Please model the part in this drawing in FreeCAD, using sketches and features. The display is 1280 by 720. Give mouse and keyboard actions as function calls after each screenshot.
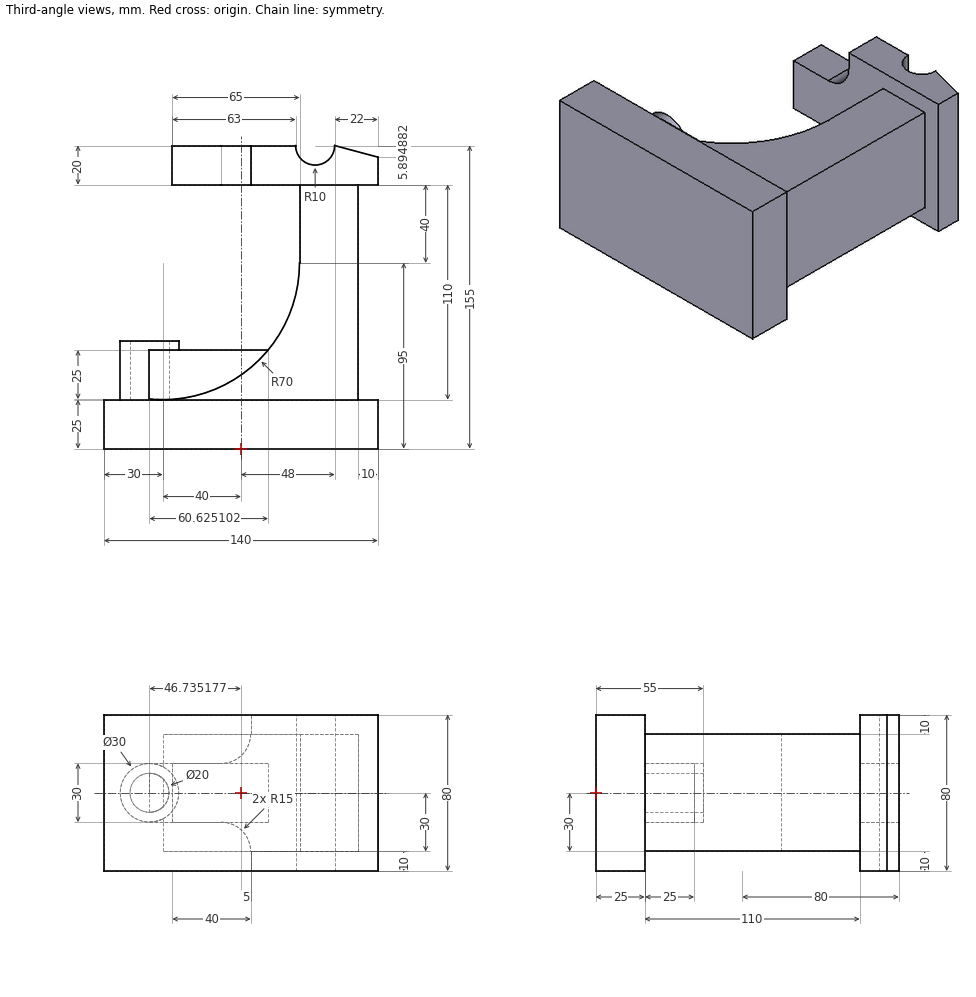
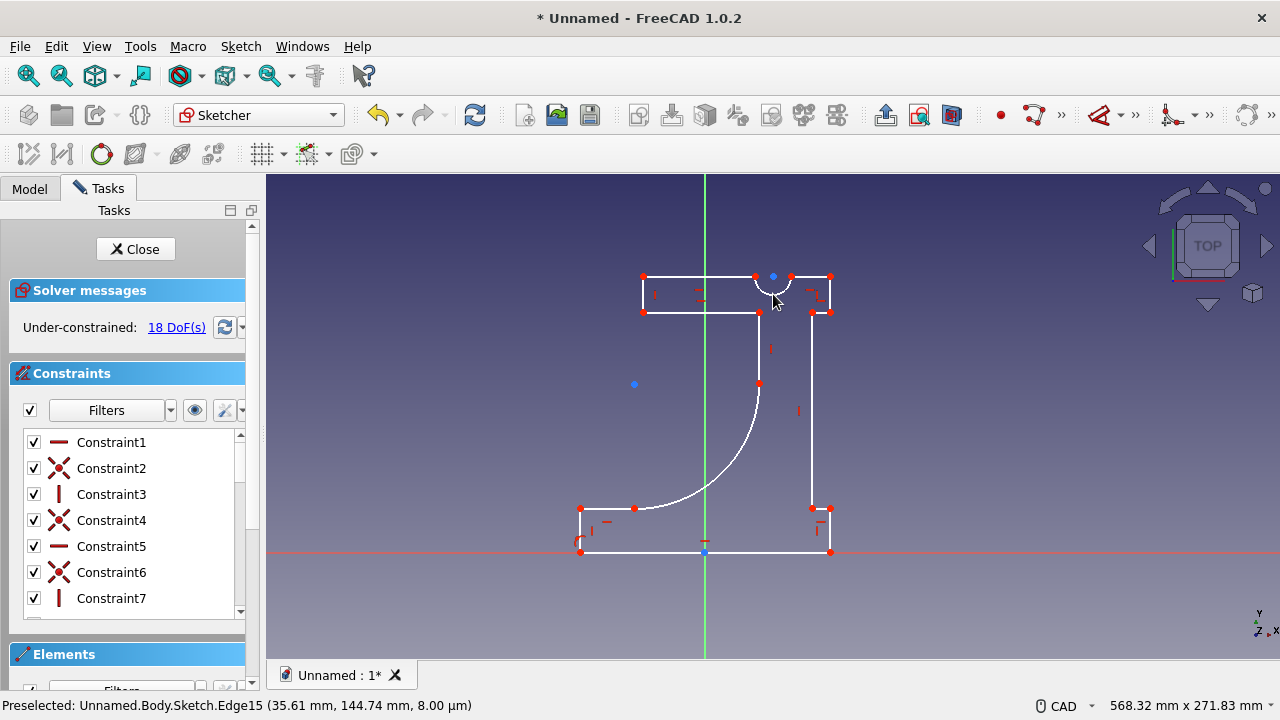
click(580, 509)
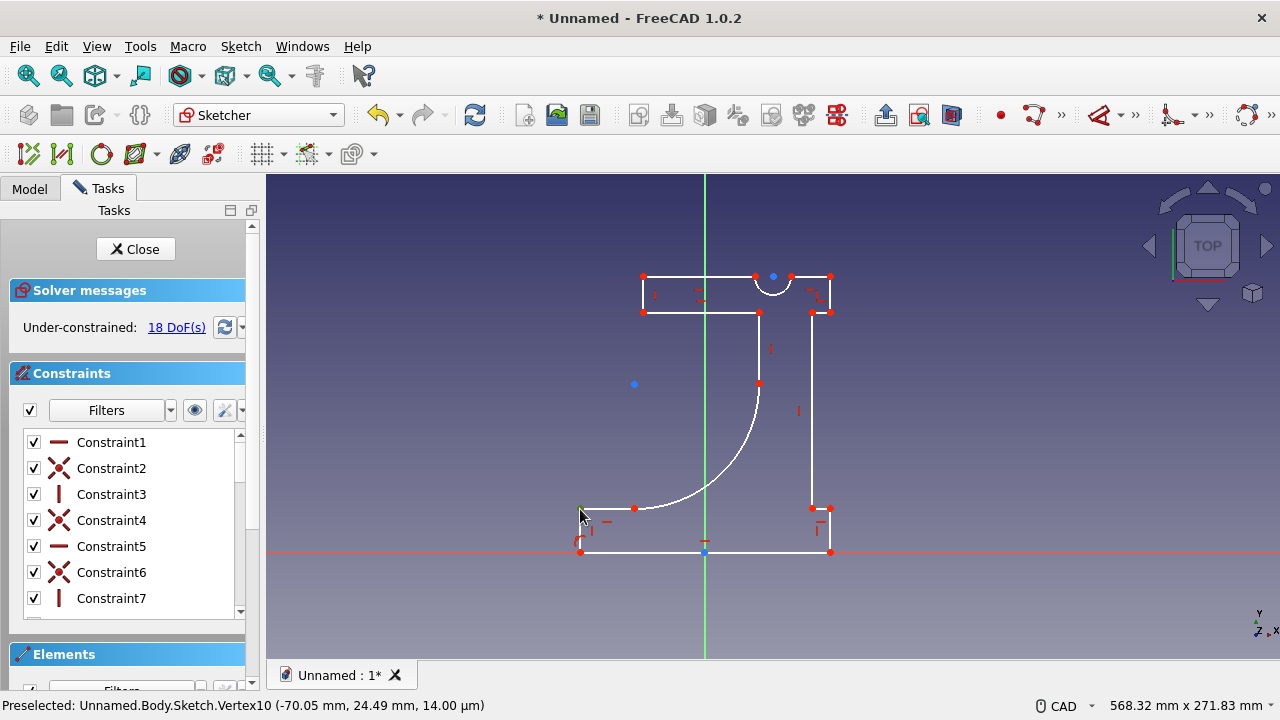
click(830, 509)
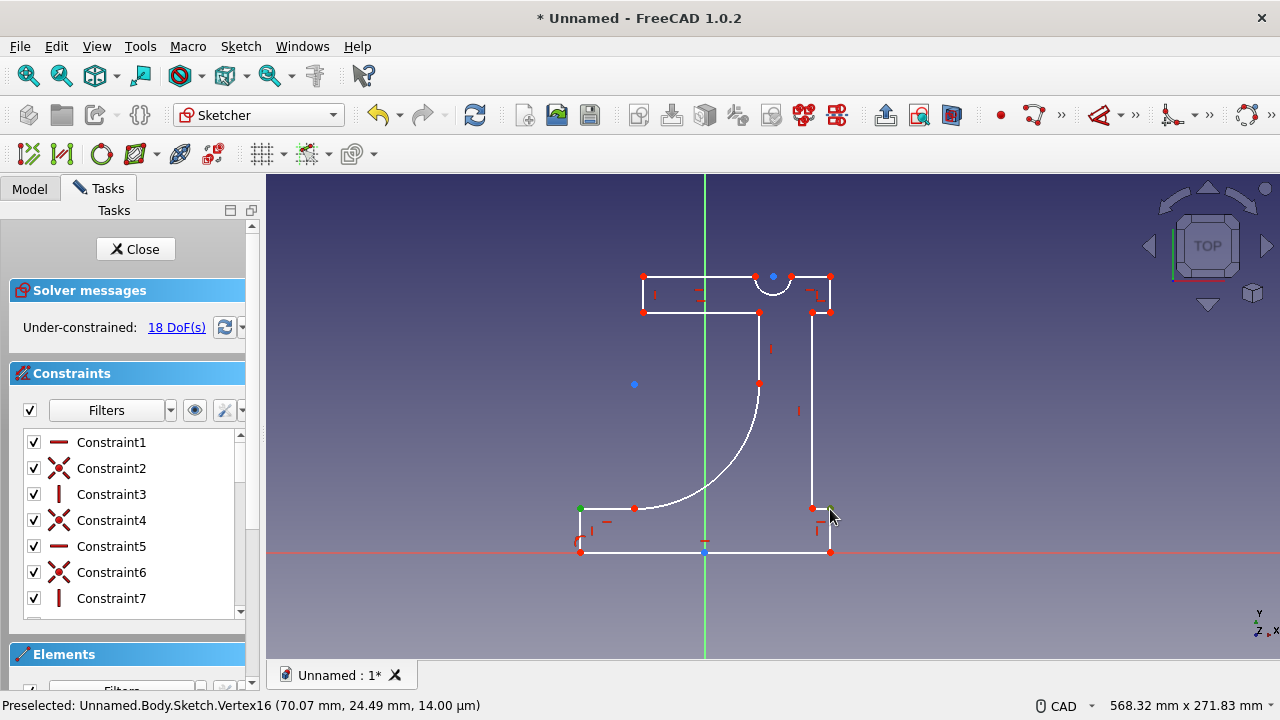
click(705, 600)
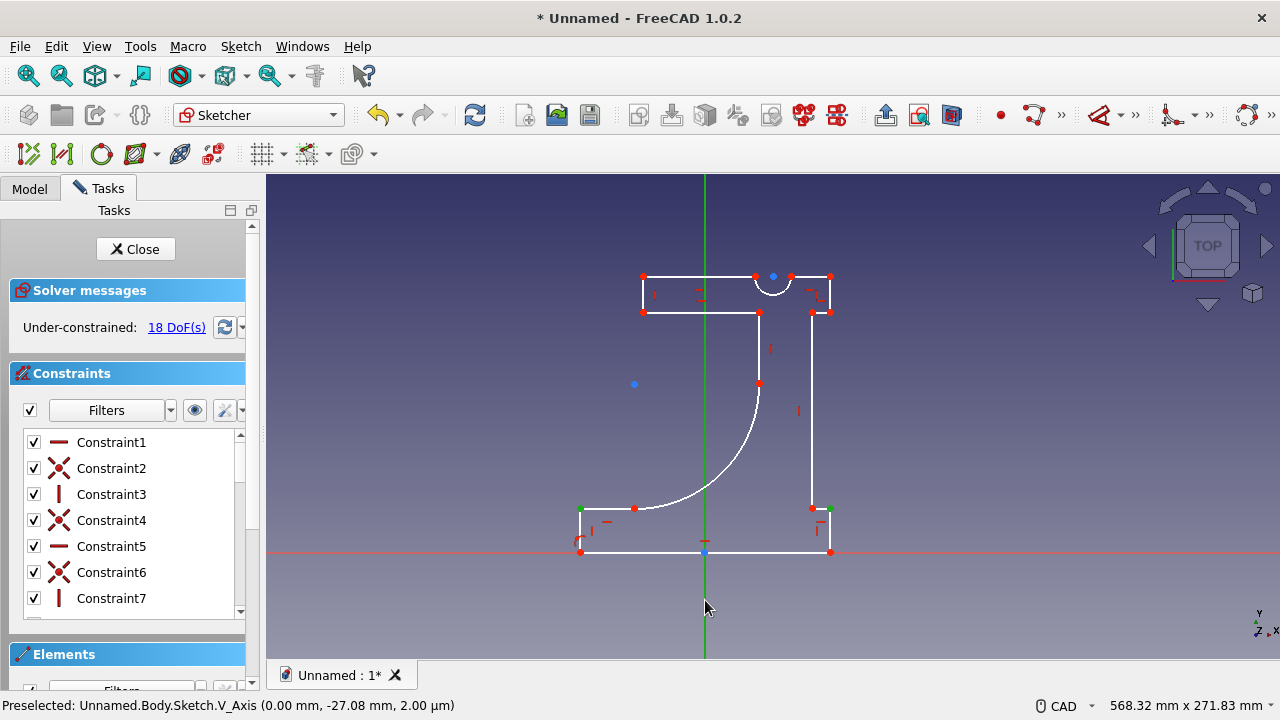
key(s)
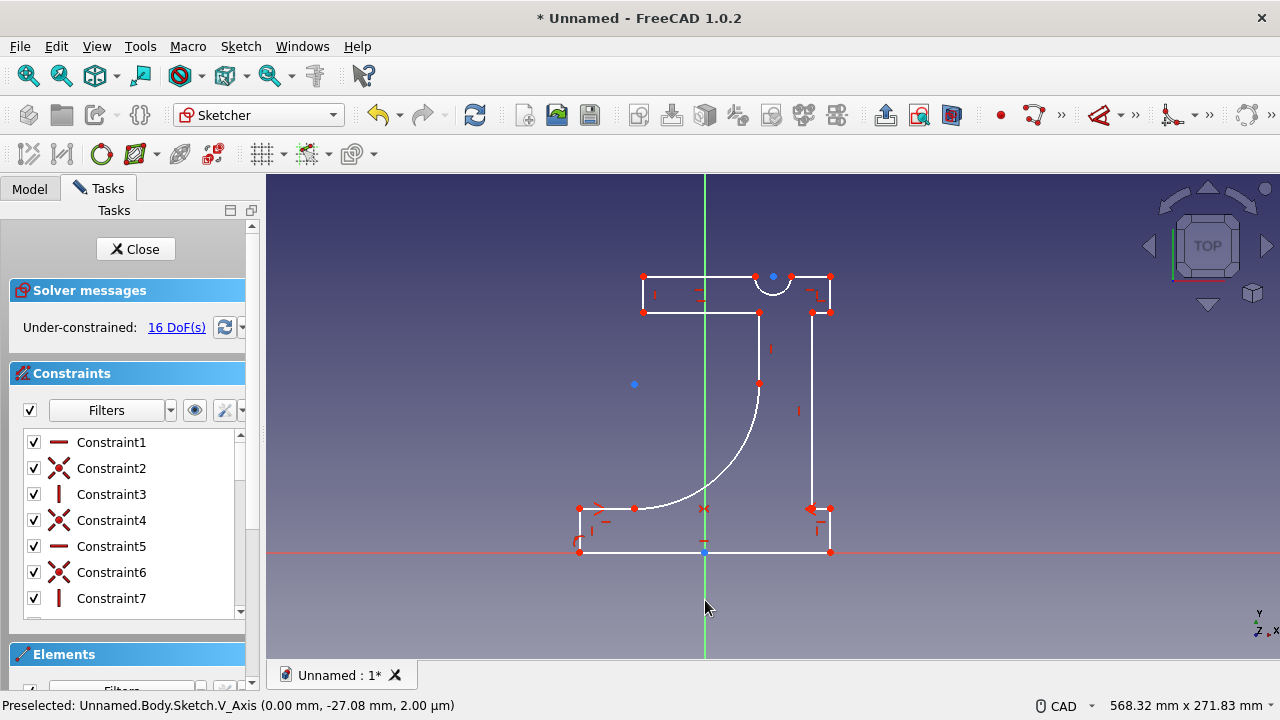
click(1098, 116)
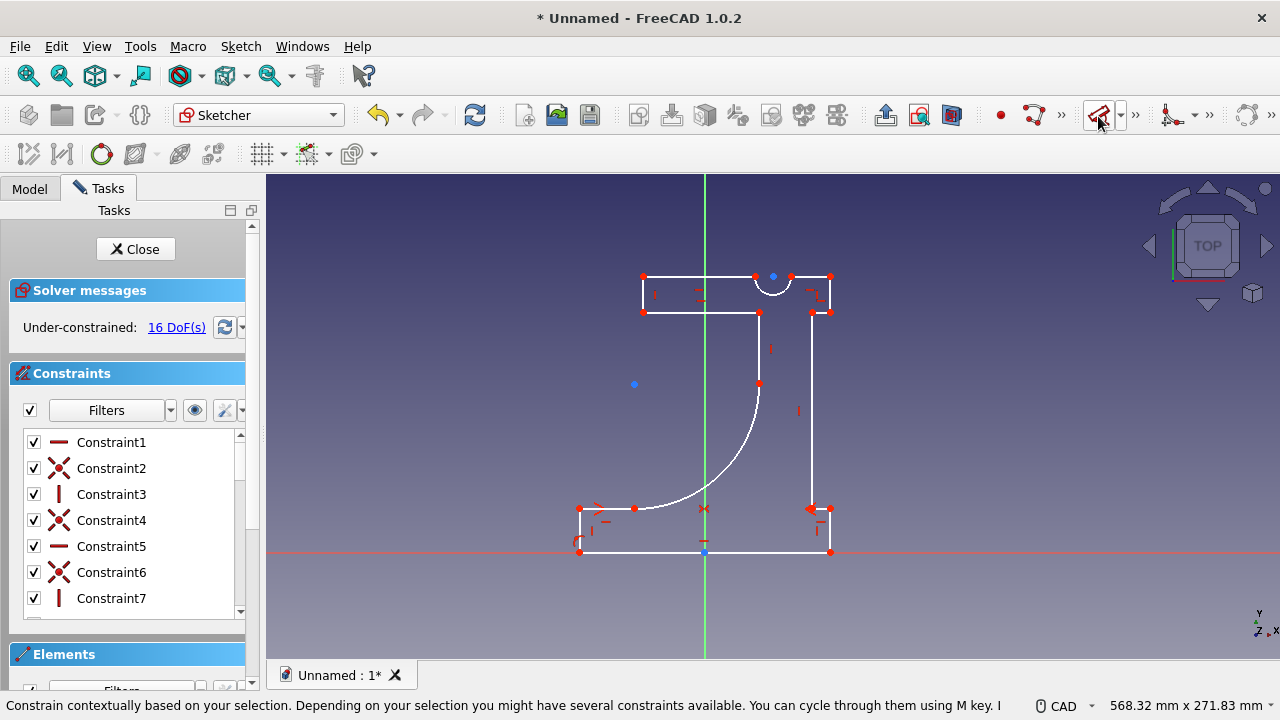
click(691, 495)
click(764, 472)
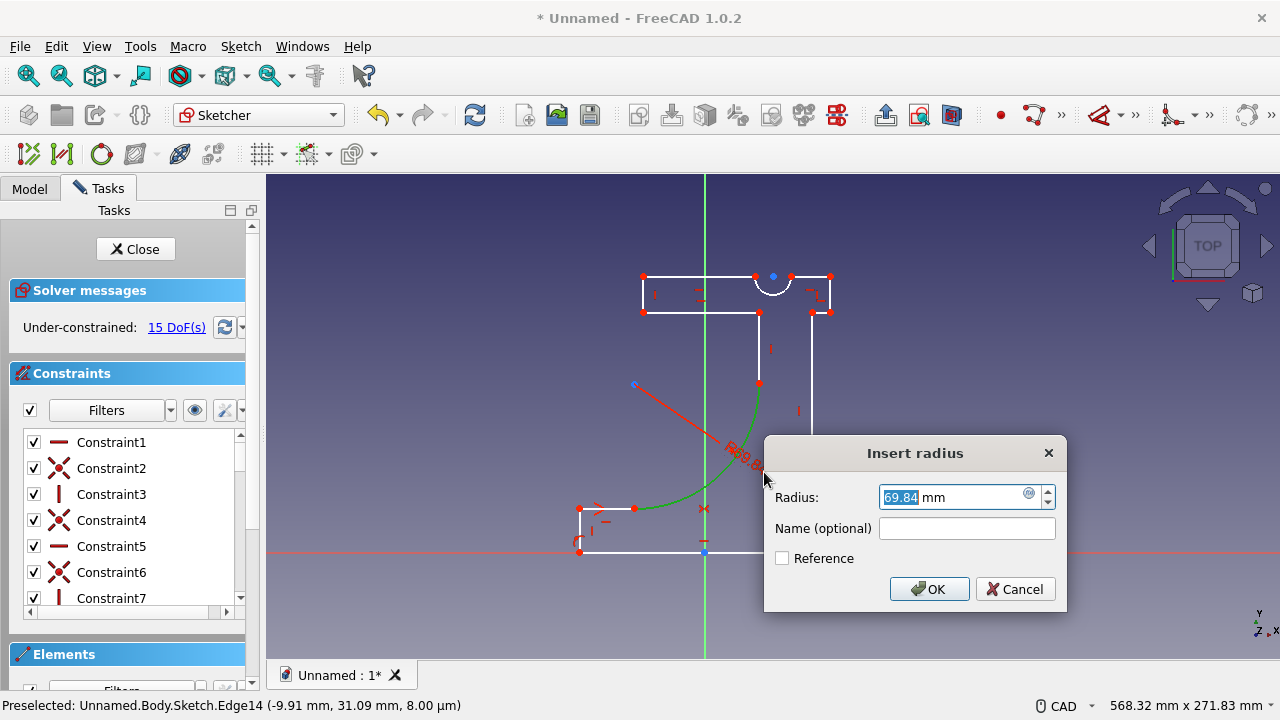
text(70)
key(Return)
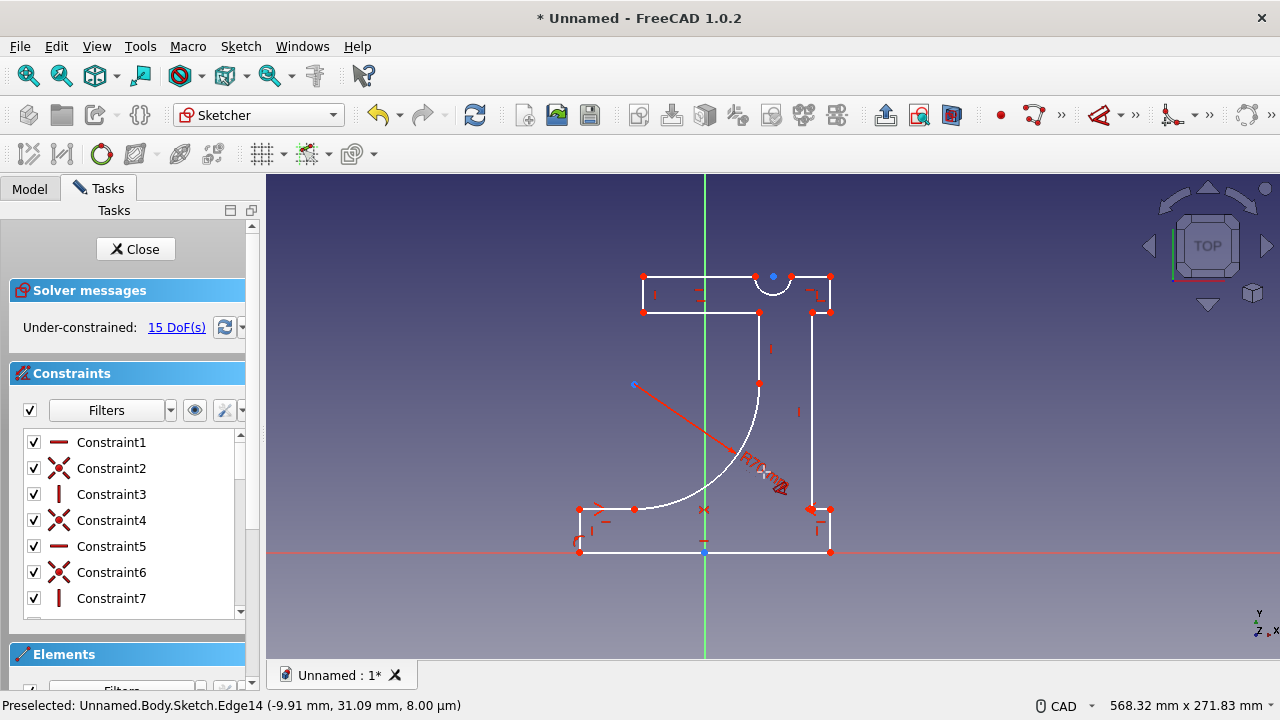
scroll(762, 292, up, 4)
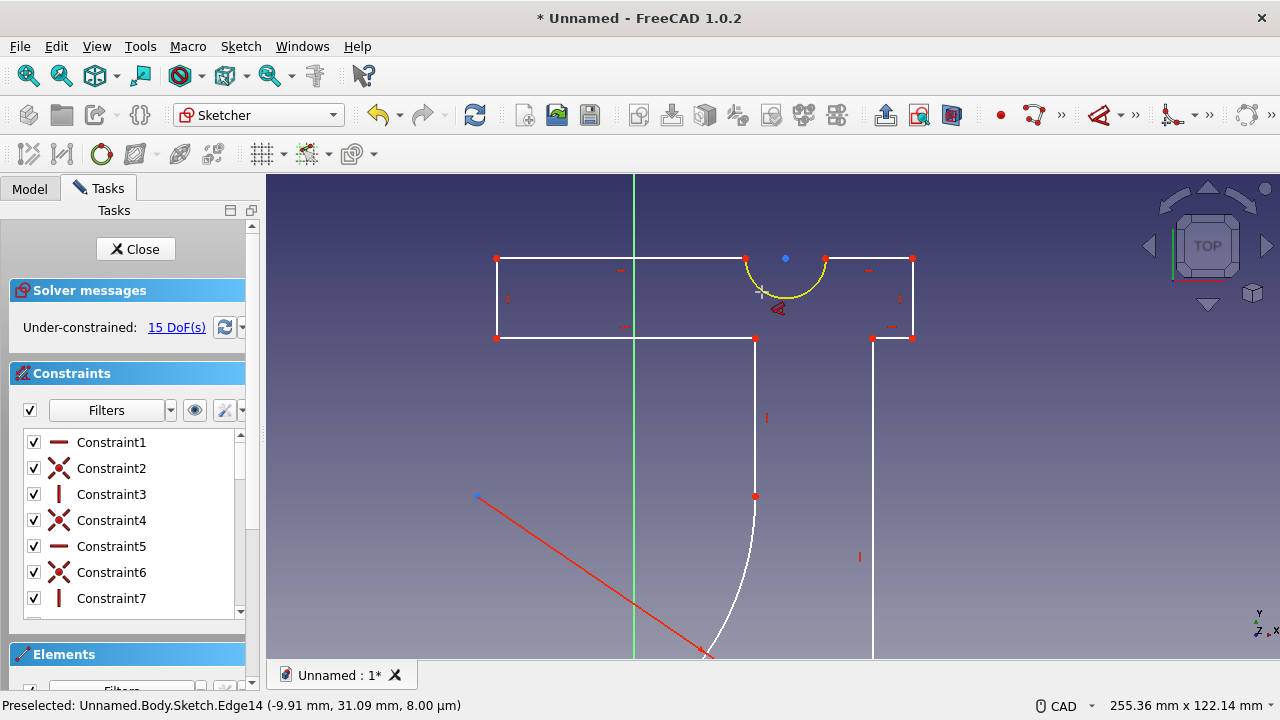
click(762, 291)
click(743, 317)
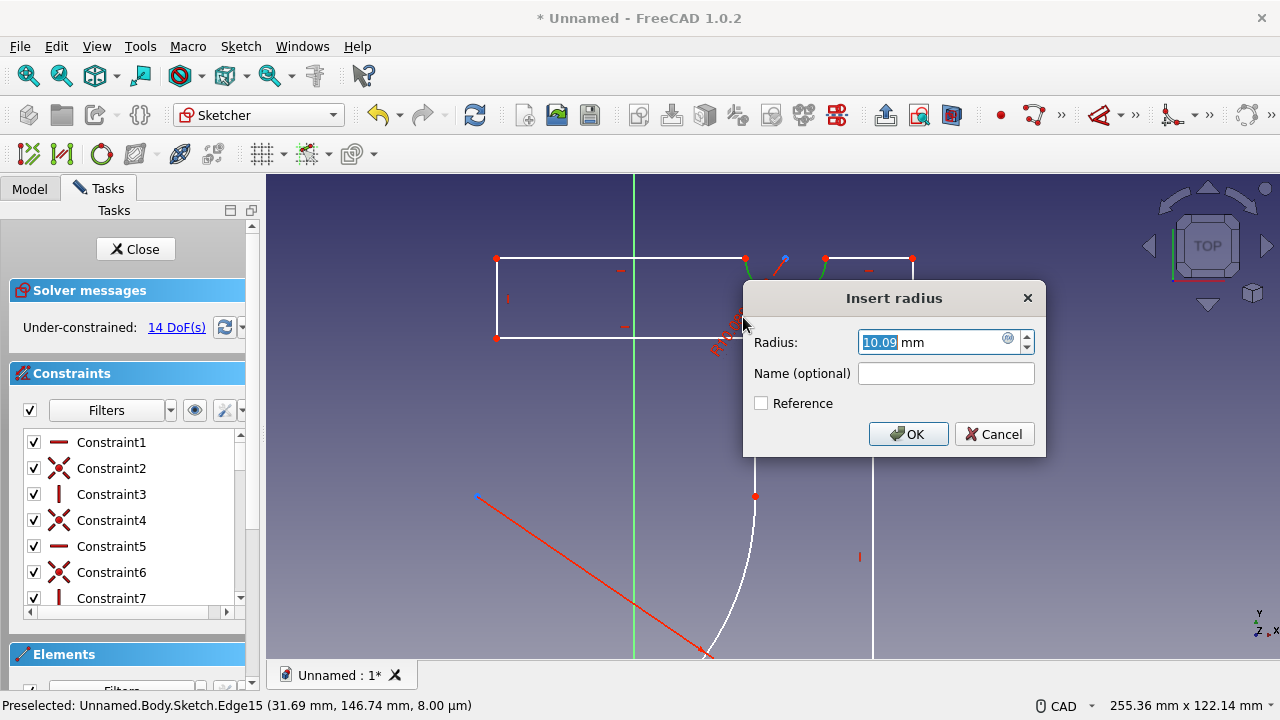
text(10)
key(Return)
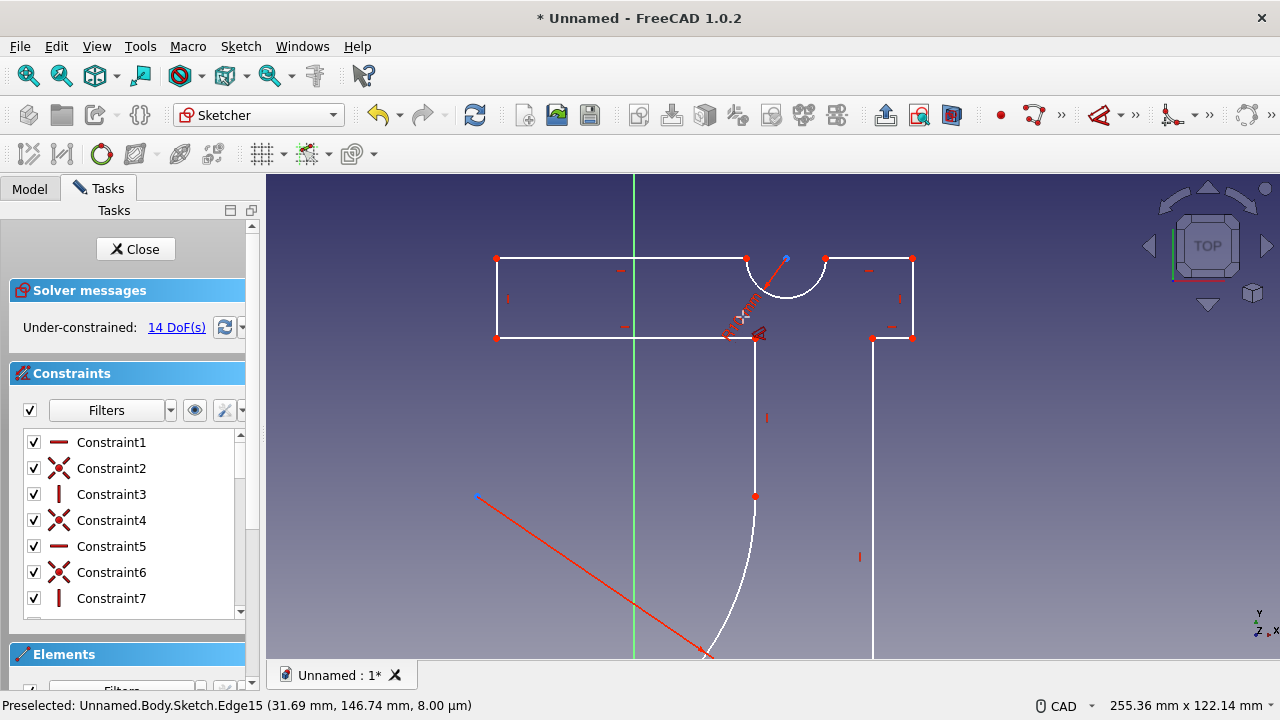
click(672, 258)
click(564, 224)